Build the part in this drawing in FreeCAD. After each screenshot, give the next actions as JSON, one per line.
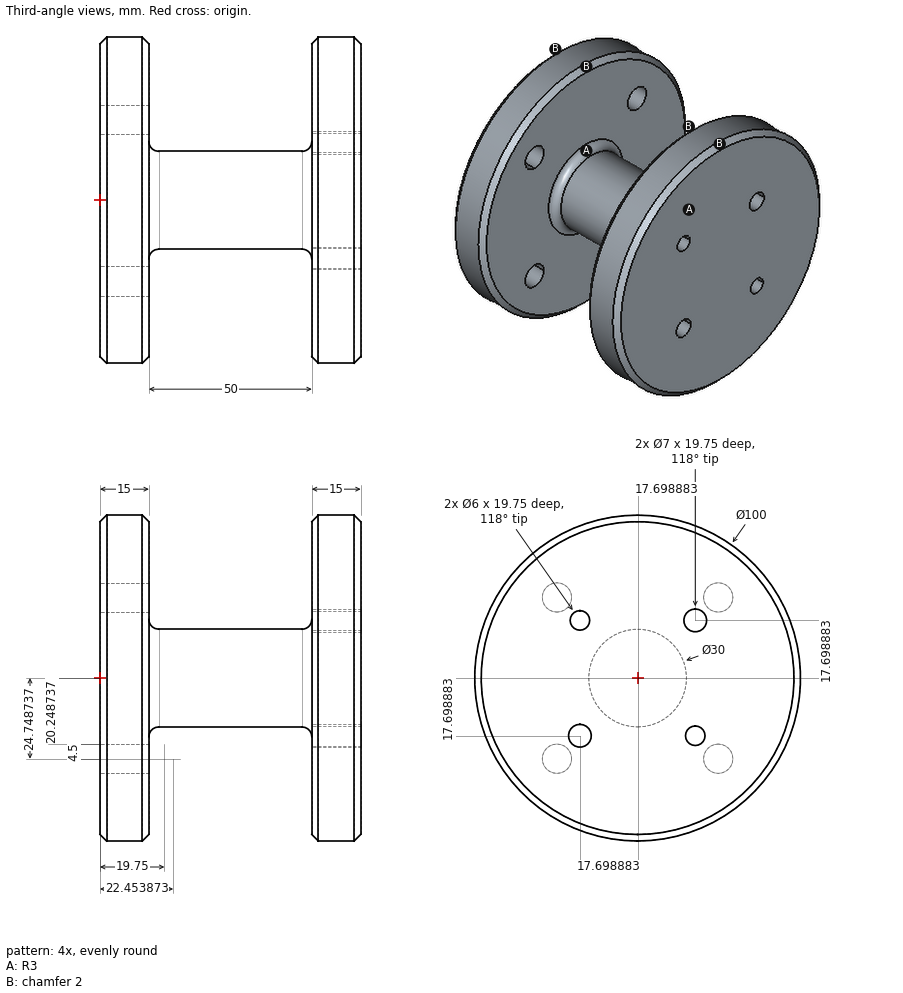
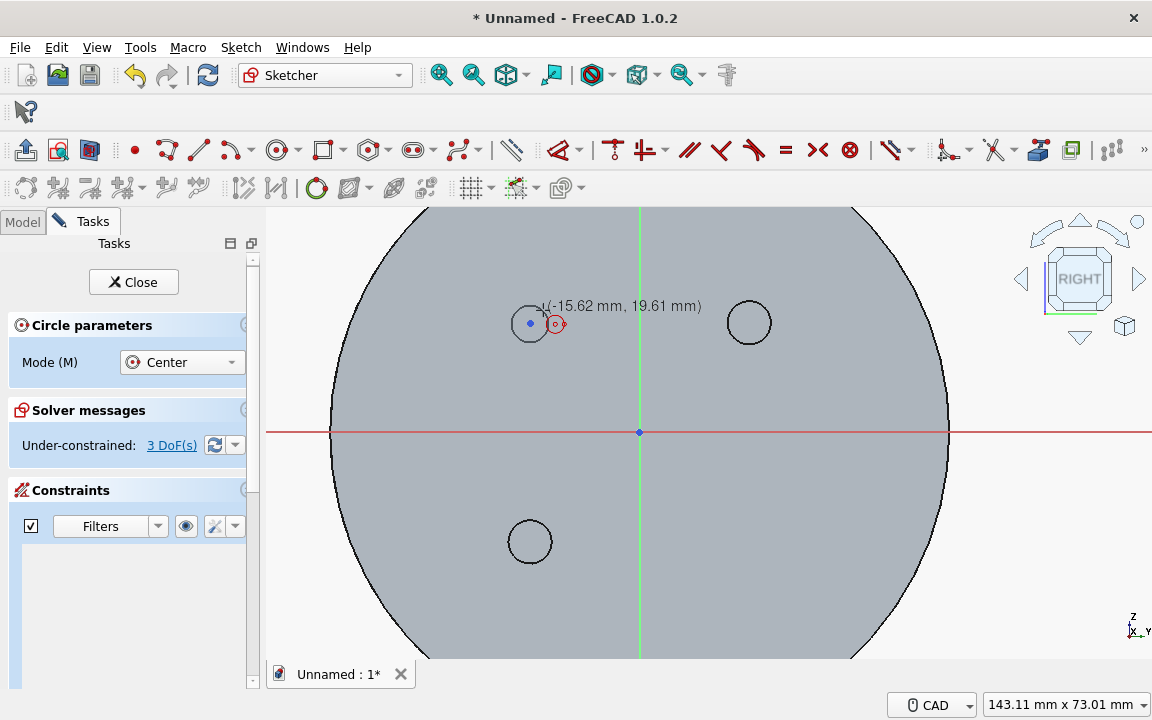
{"action": "left_click", "coordinate": [749, 542]}
{"action": "left_click", "coordinate": [762, 529]}
{"action": "key", "text": "Escape"}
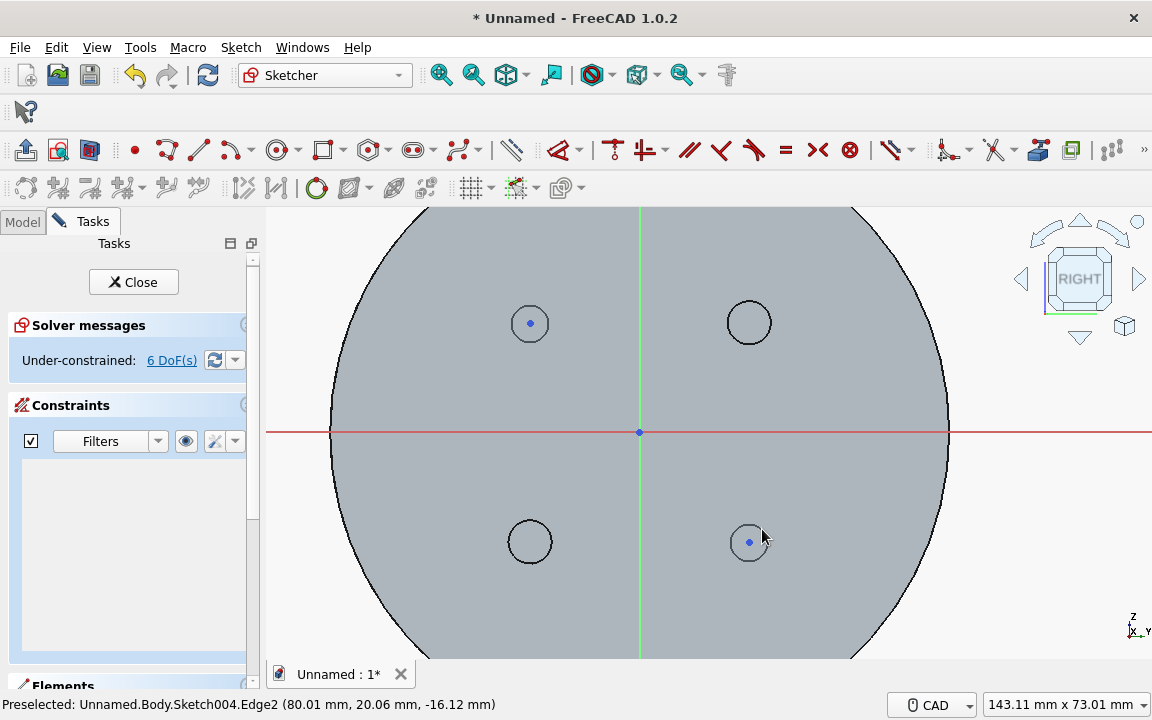
{"action": "left_click", "coordinate": [543, 311]}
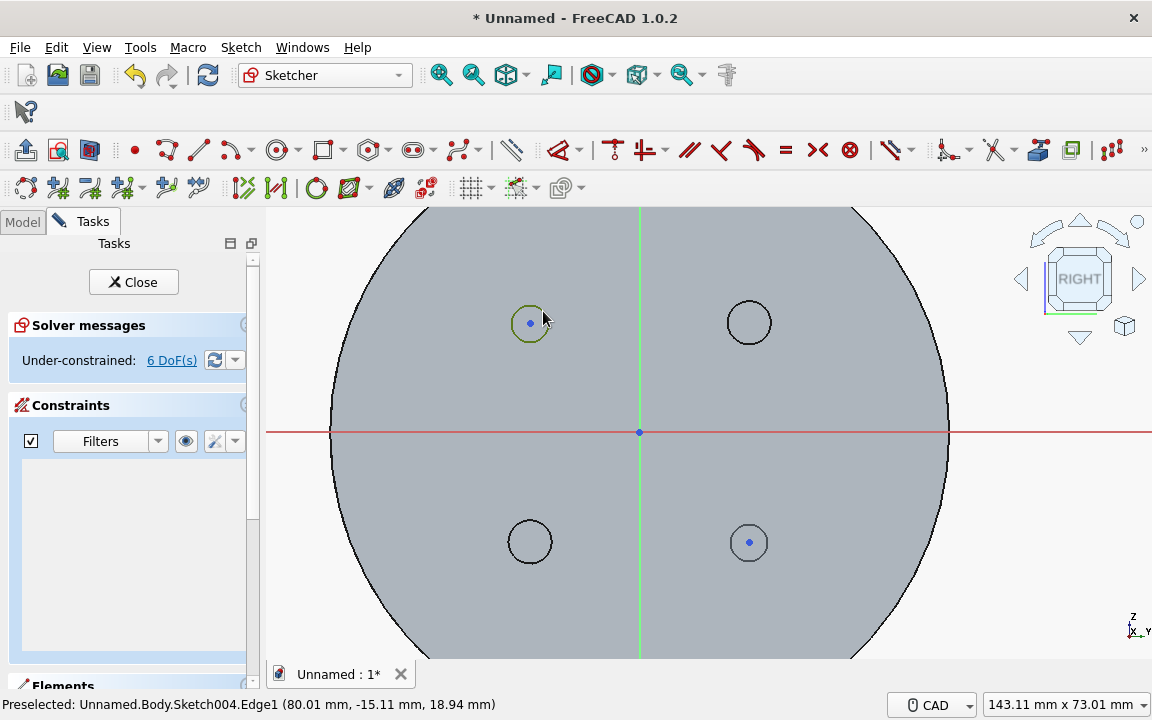
{"action": "left_click", "coordinate": [762, 530]}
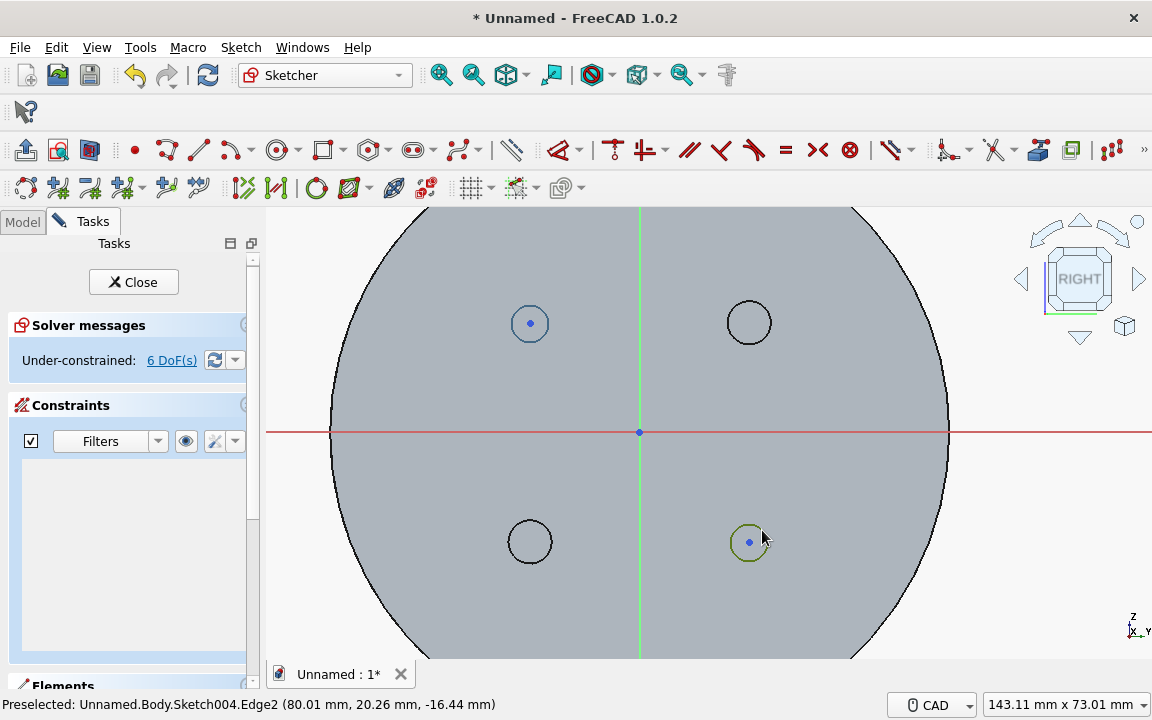
{"action": "key", "text": "e"}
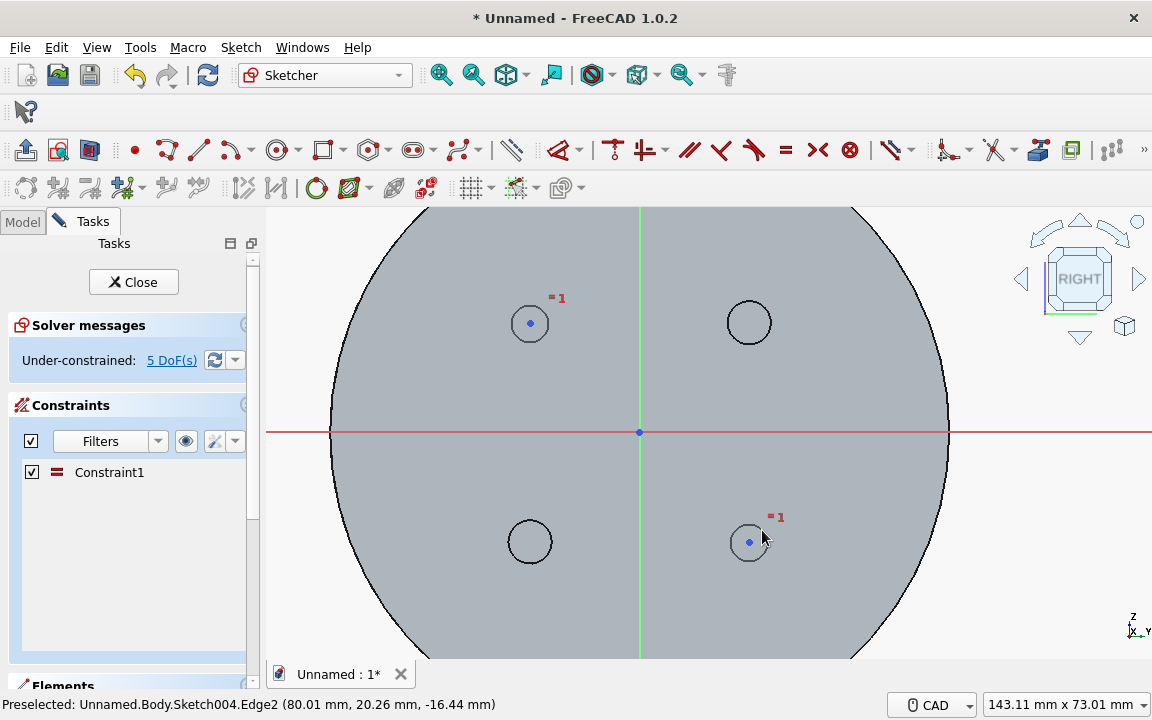
{"action": "left_click", "coordinate": [558, 150]}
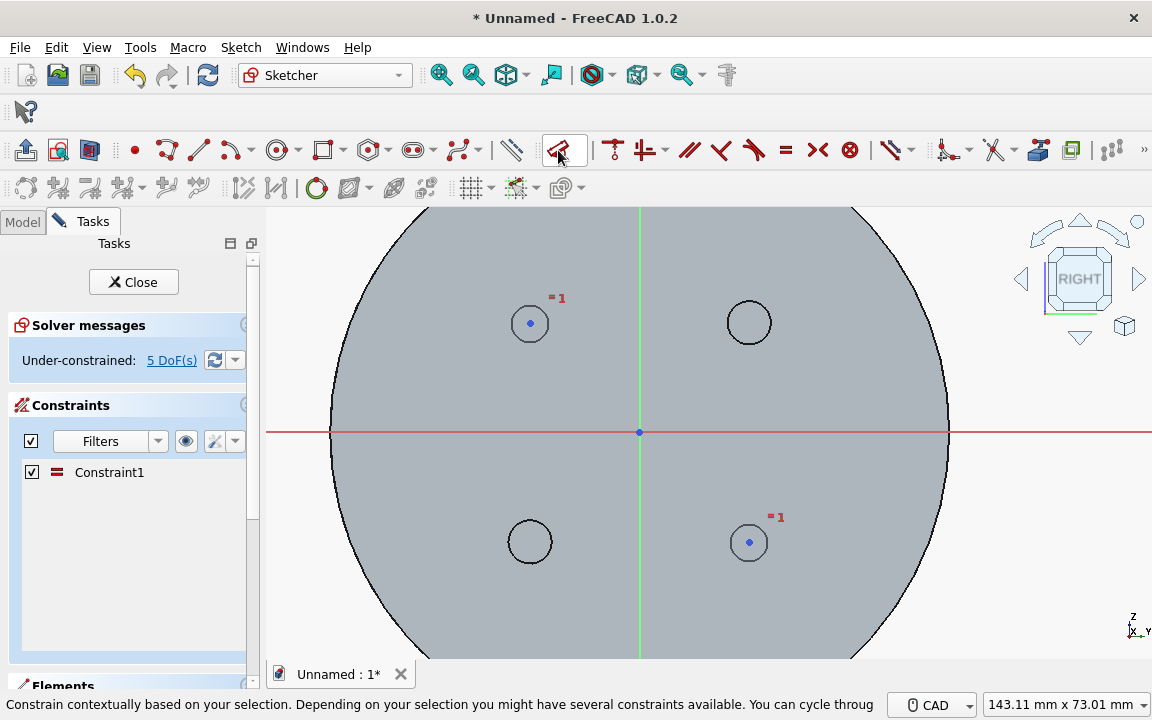
{"action": "left_click", "coordinate": [543, 311]}
{"action": "left_click", "coordinate": [566, 288]}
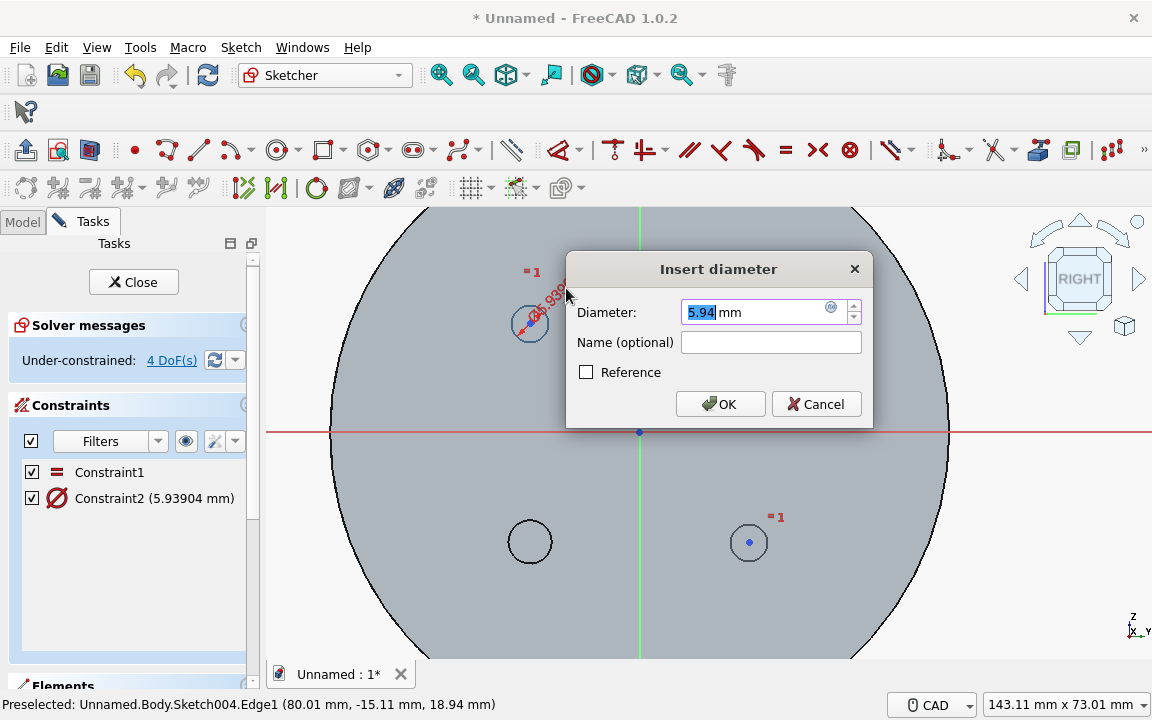
{"action": "type", "text": "6"}
{"action": "key", "text": "Return"}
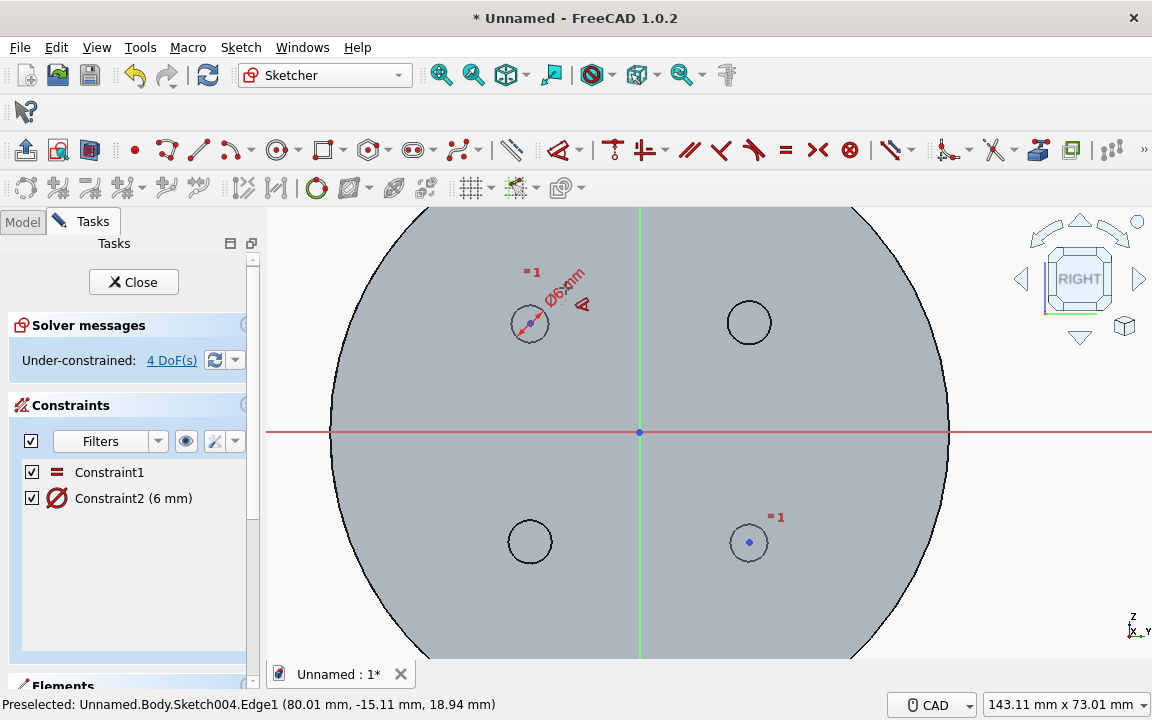
{"action": "left_click", "coordinate": [530, 324]}
{"action": "left_click", "coordinate": [585, 466]}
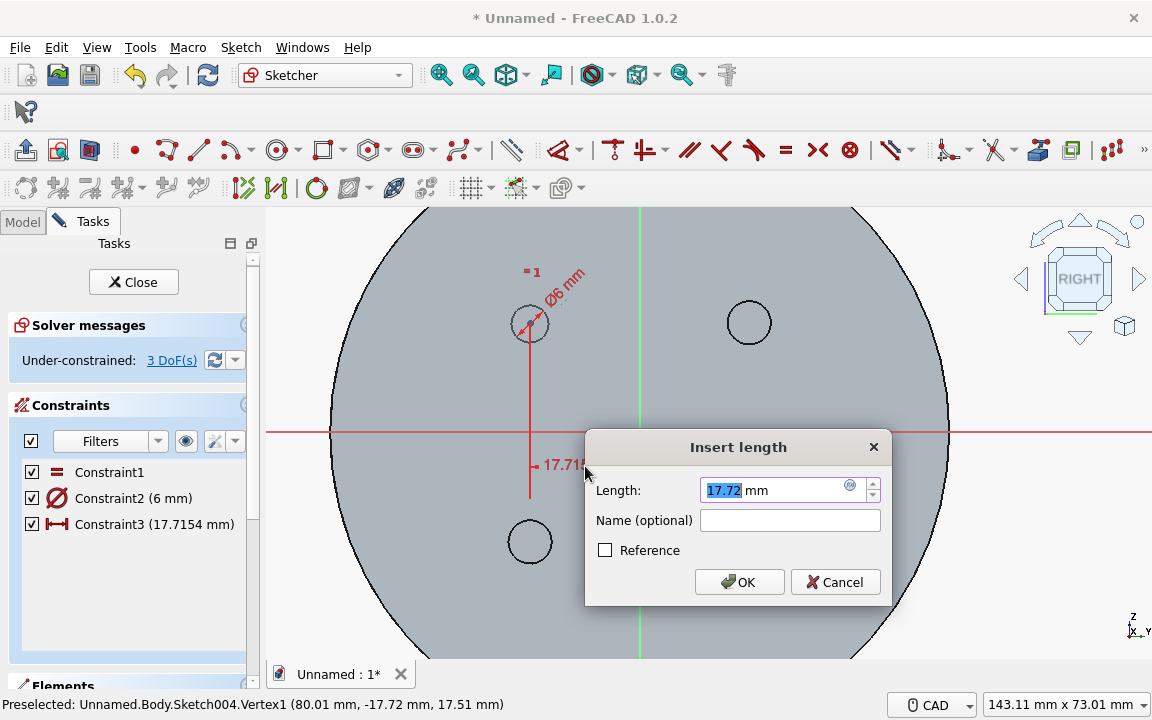
{"action": "type", "text": "17.698883"}
{"action": "key", "text": "Return"}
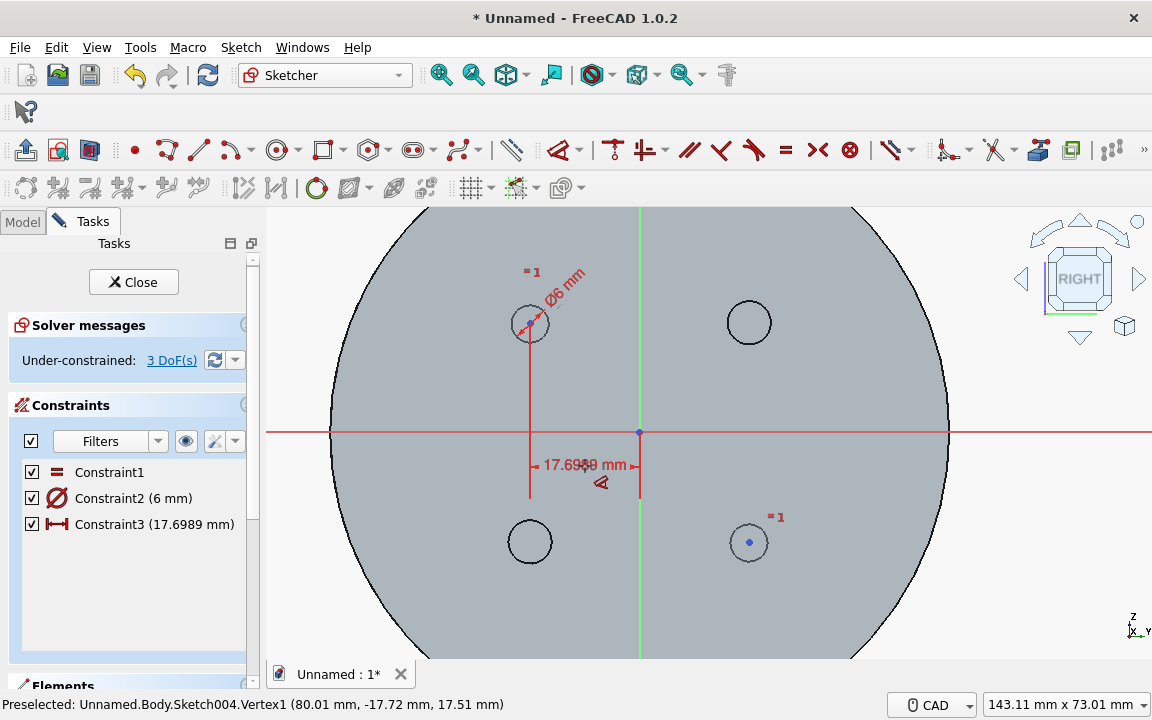
{"action": "left_click", "coordinate": [530, 324]}
{"action": "left_click", "coordinate": [496, 378]}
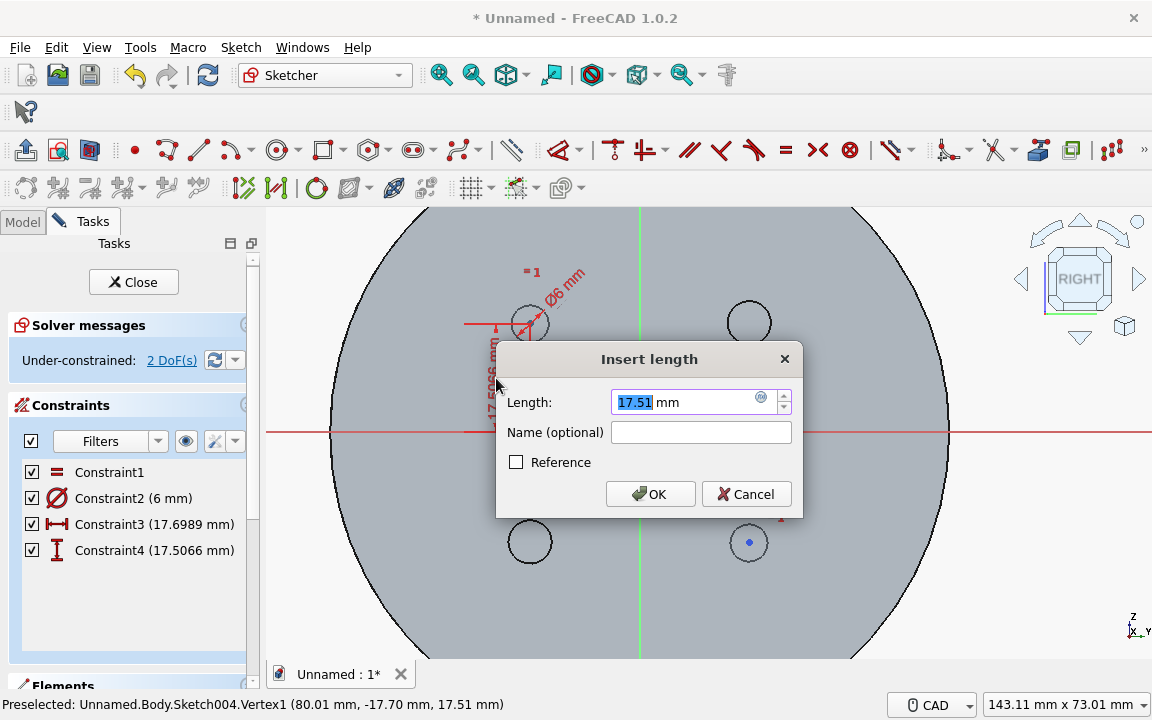
{"action": "type", "text": "17.698883"}
{"action": "key", "text": "Return"}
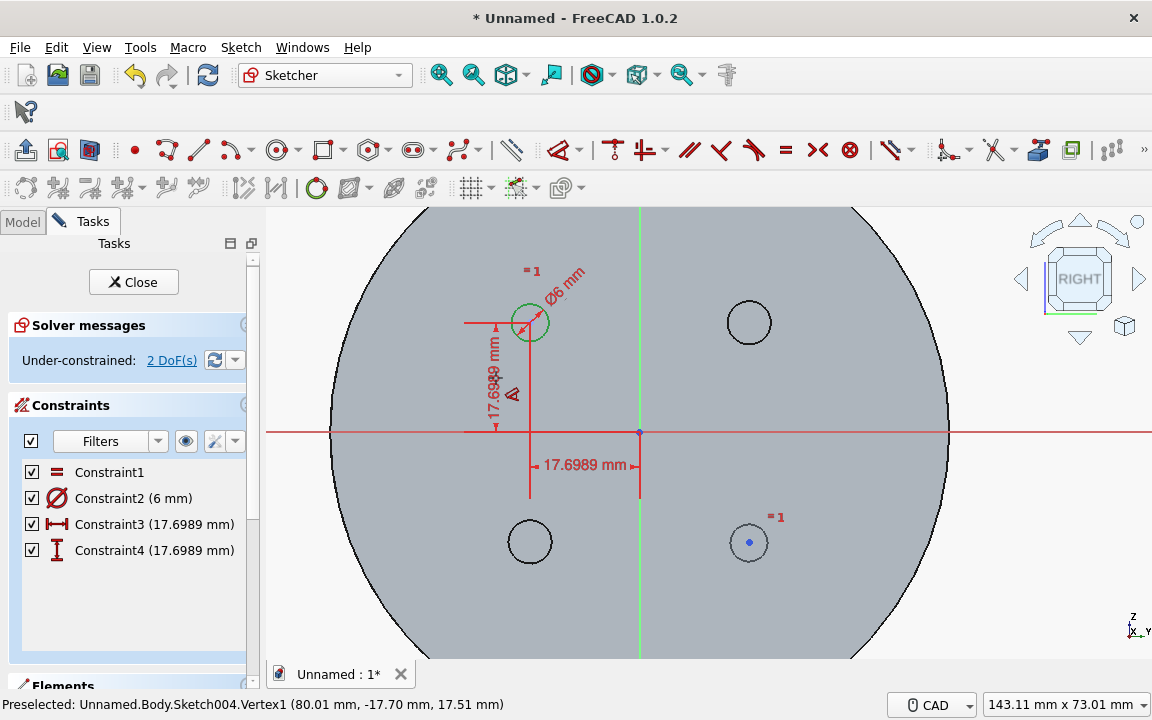
{"action": "left_click", "coordinate": [749, 543]}
{"action": "left_click", "coordinate": [694, 577]}